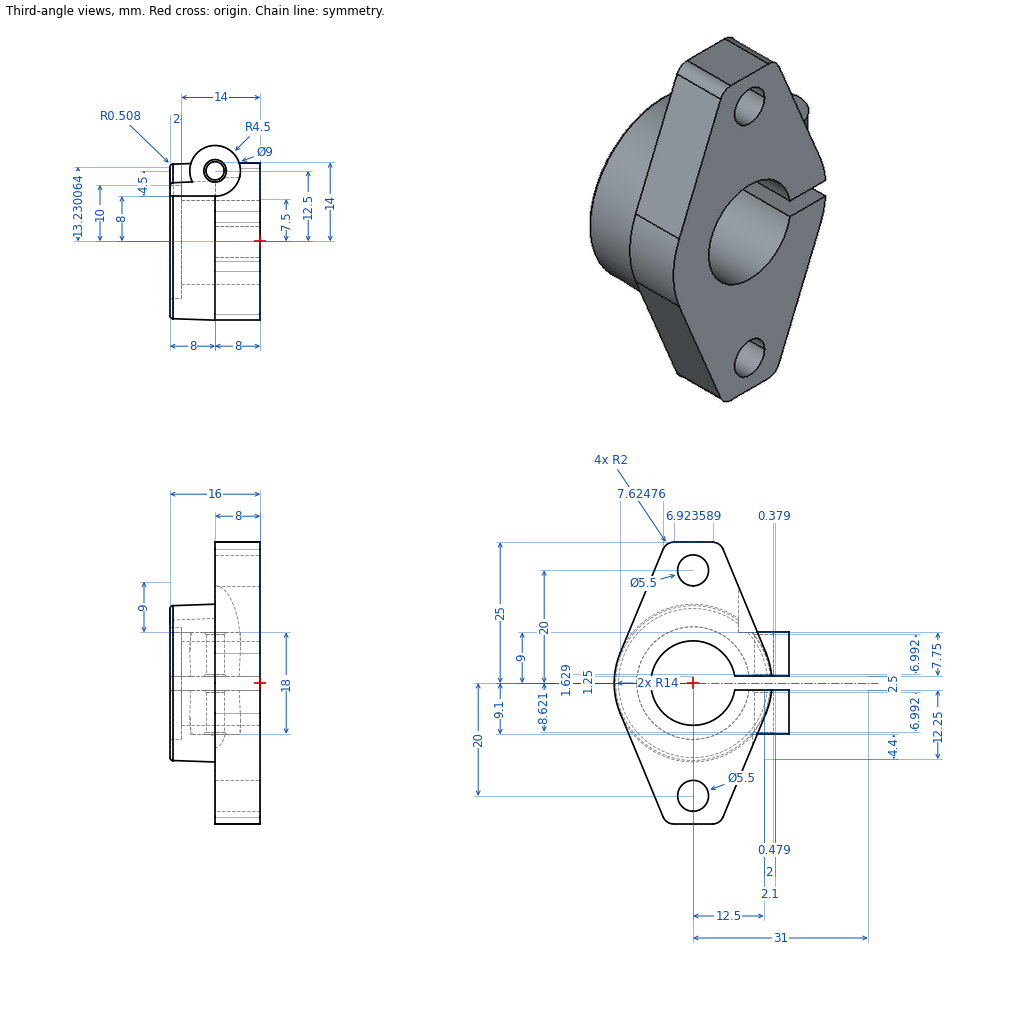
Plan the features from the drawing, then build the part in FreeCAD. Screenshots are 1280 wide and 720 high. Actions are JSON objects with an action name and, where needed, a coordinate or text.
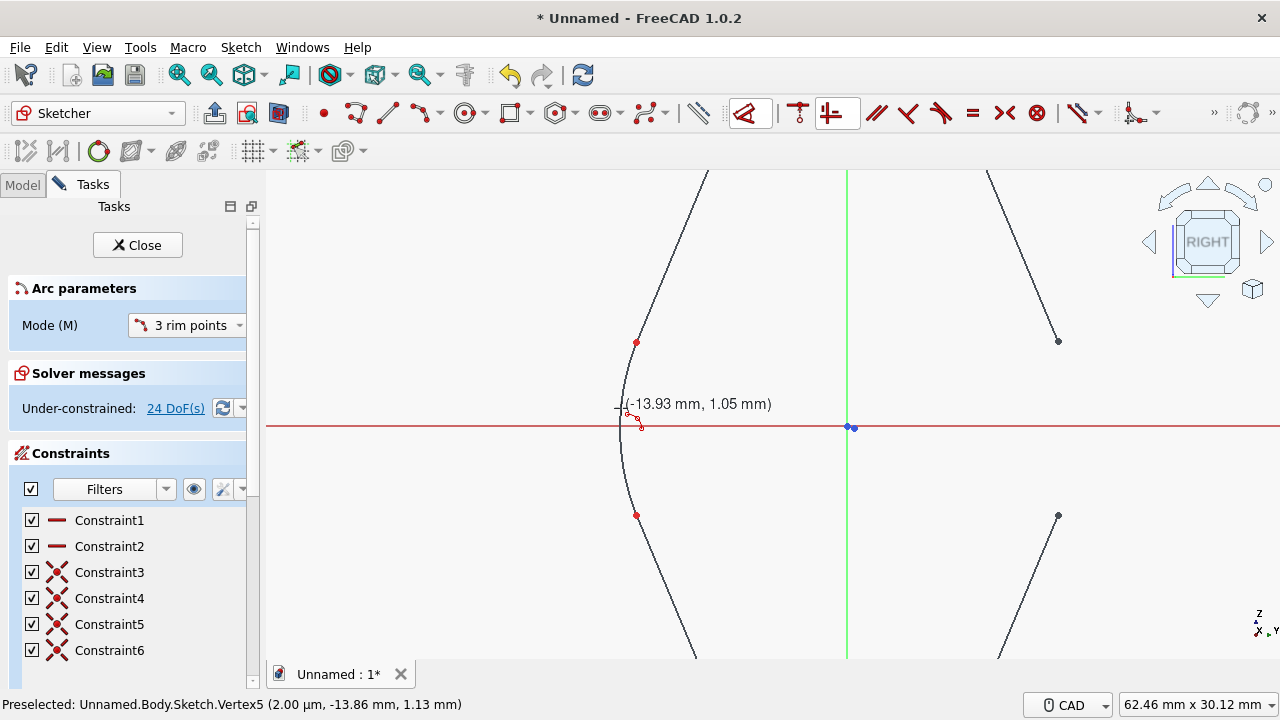
{"action": "scroll", "coordinate": [621, 408], "scroll_direction": "down", "scroll_amount": 5}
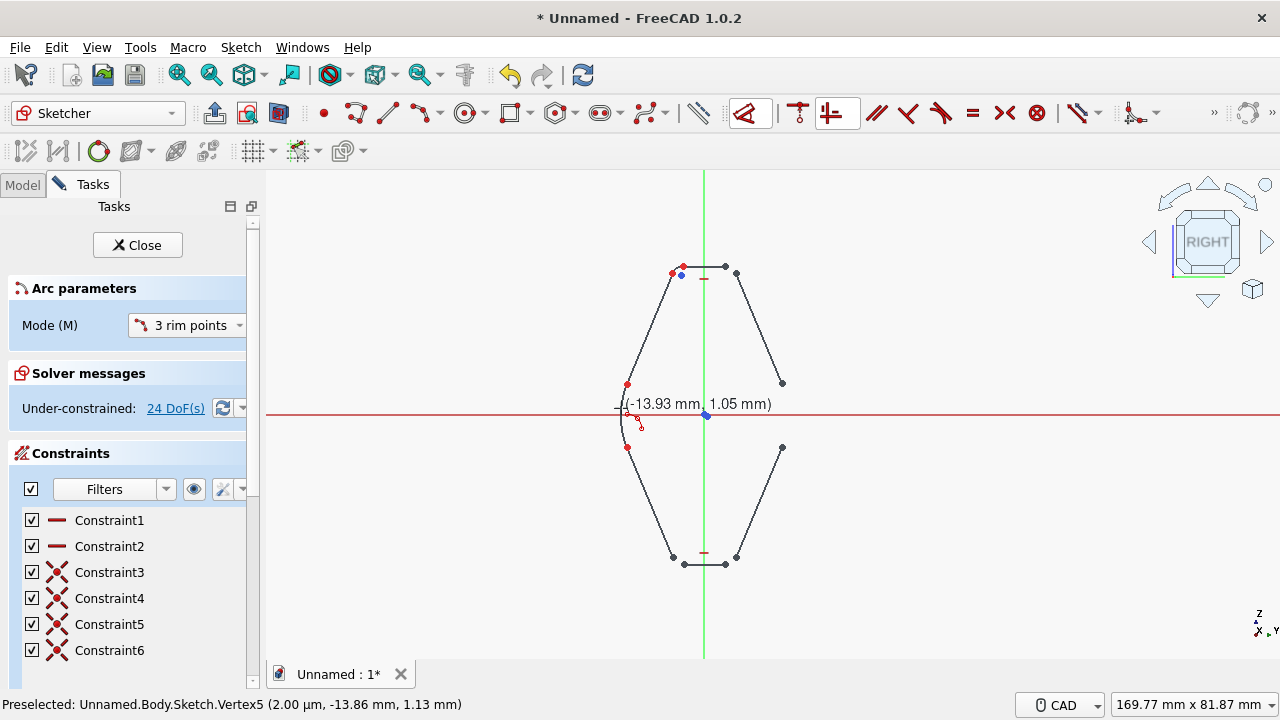
{"action": "left_click", "coordinate": [673, 558]}
{"action": "left_click", "coordinate": [684, 565]}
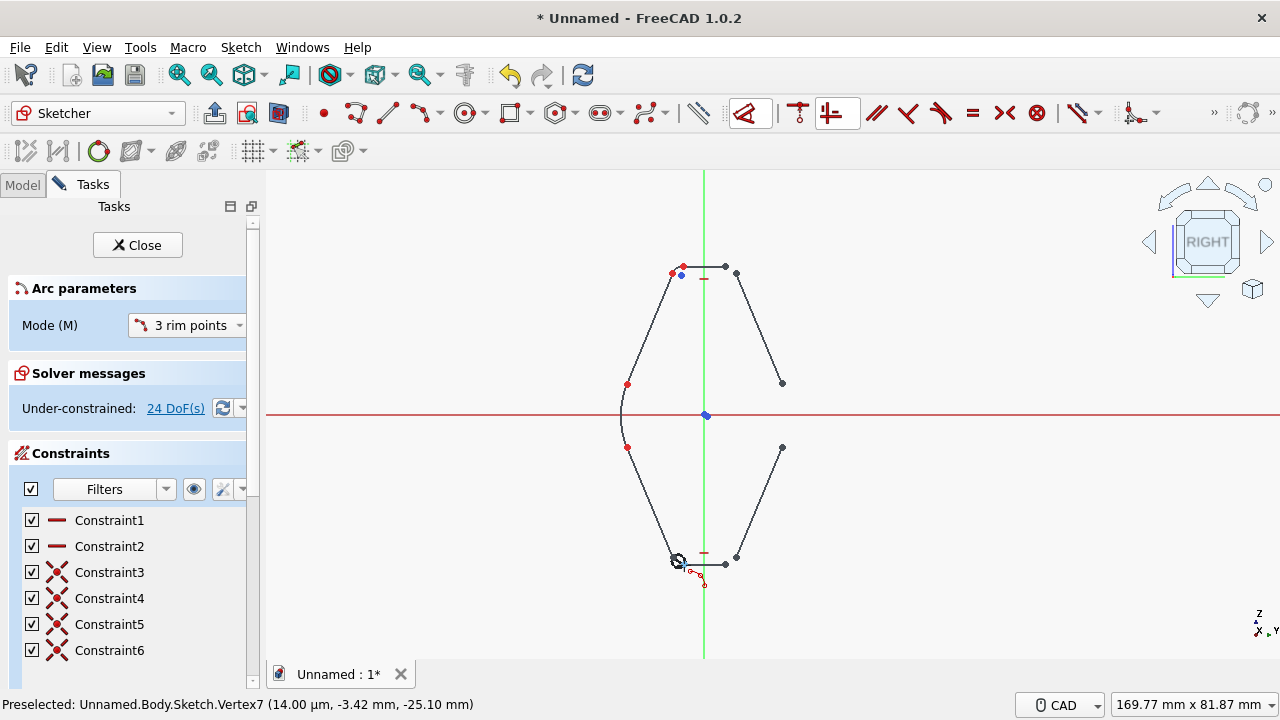
{"action": "scroll", "coordinate": [677, 562], "scroll_direction": "up", "scroll_amount": 11}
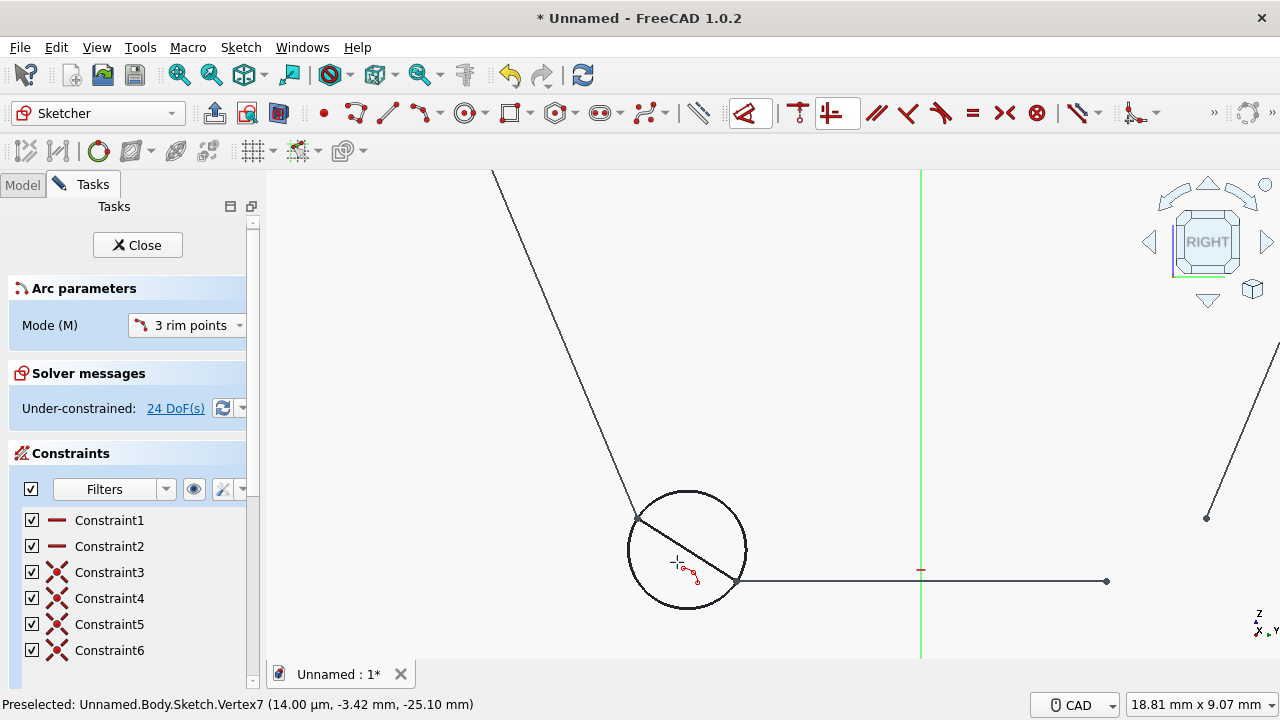
{"action": "left_click", "coordinate": [675, 558]}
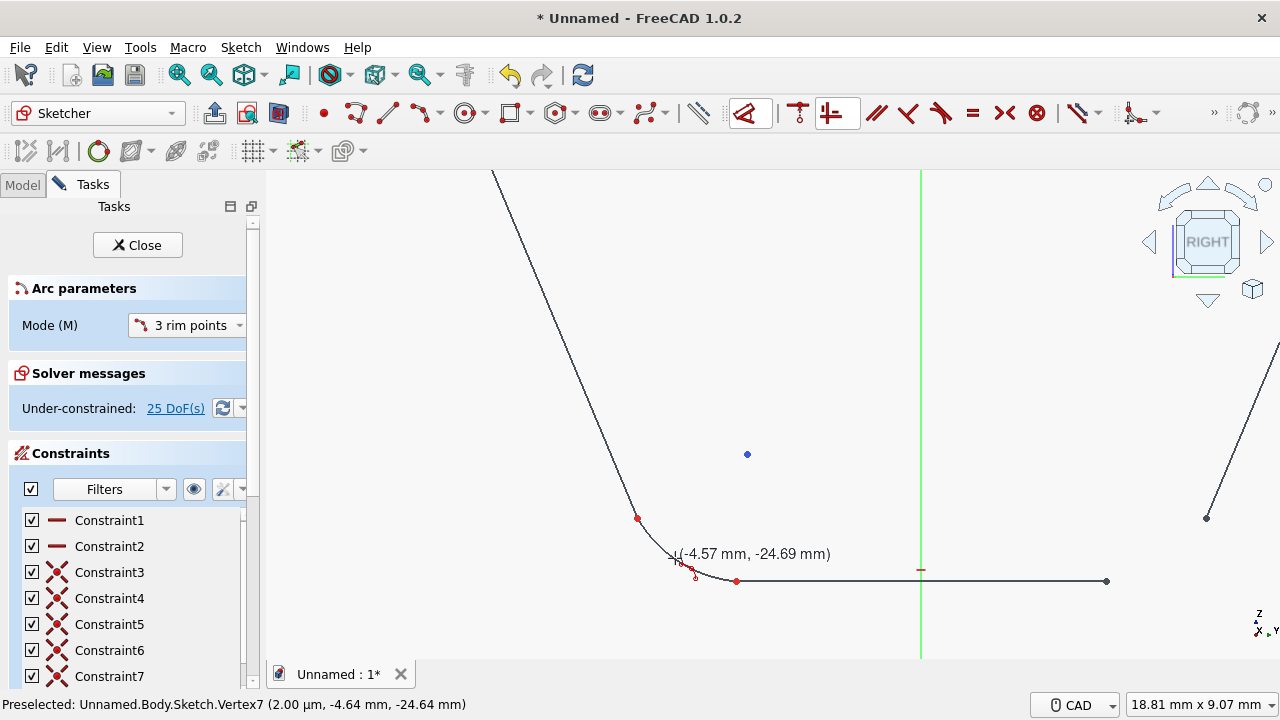
{"action": "scroll", "coordinate": [677, 562], "scroll_direction": "down", "scroll_amount": 11}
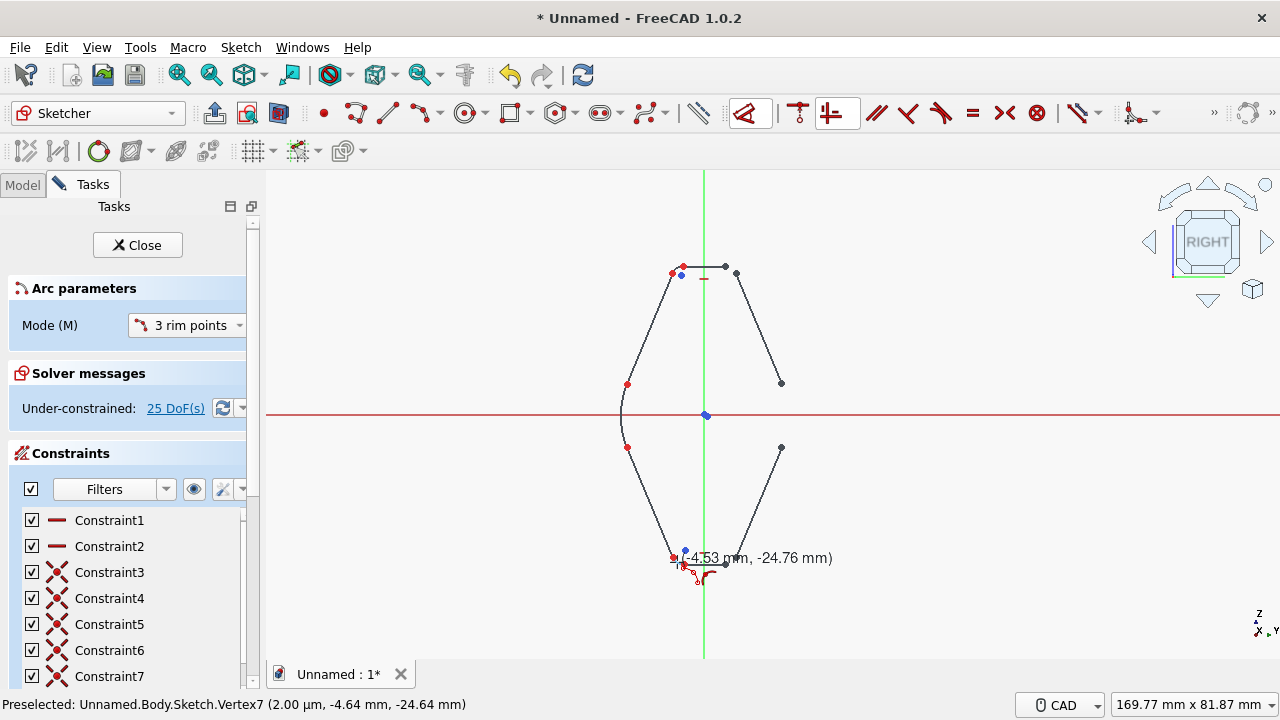
{"action": "left_click", "coordinate": [725, 565]}
{"action": "left_click", "coordinate": [736, 558]}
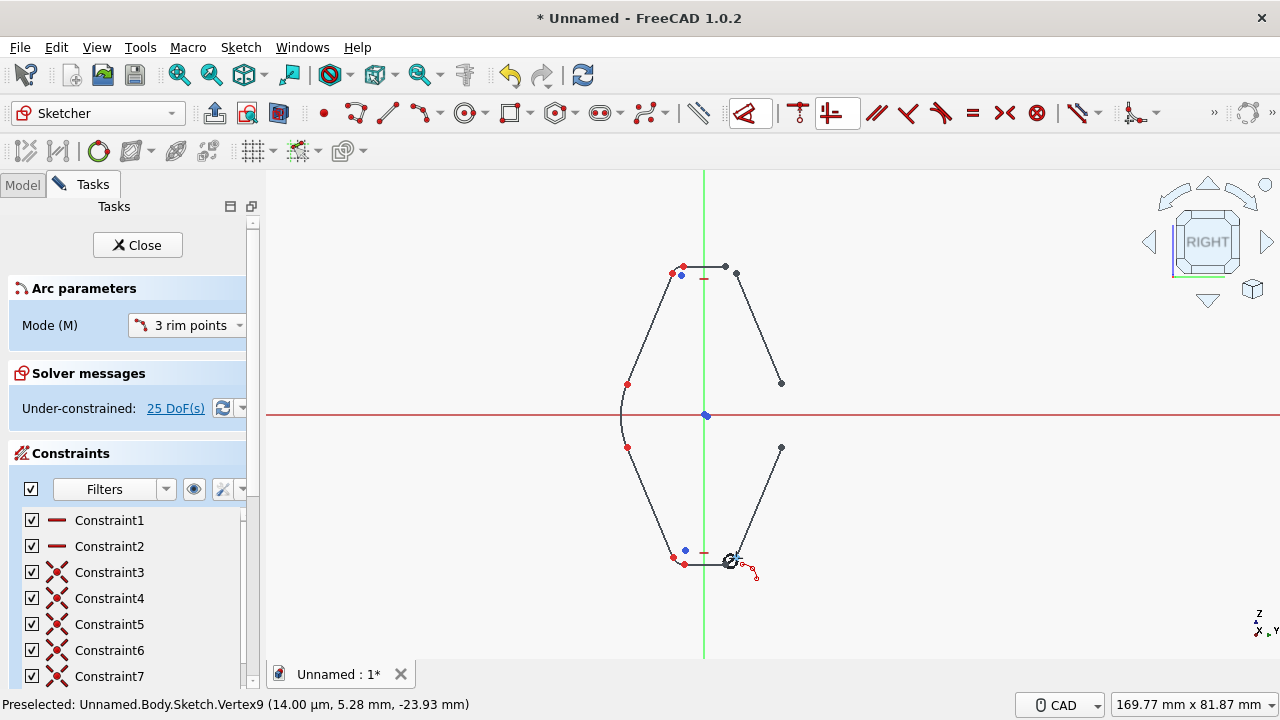
{"action": "scroll", "coordinate": [732, 562], "scroll_direction": "up", "scroll_amount": 11}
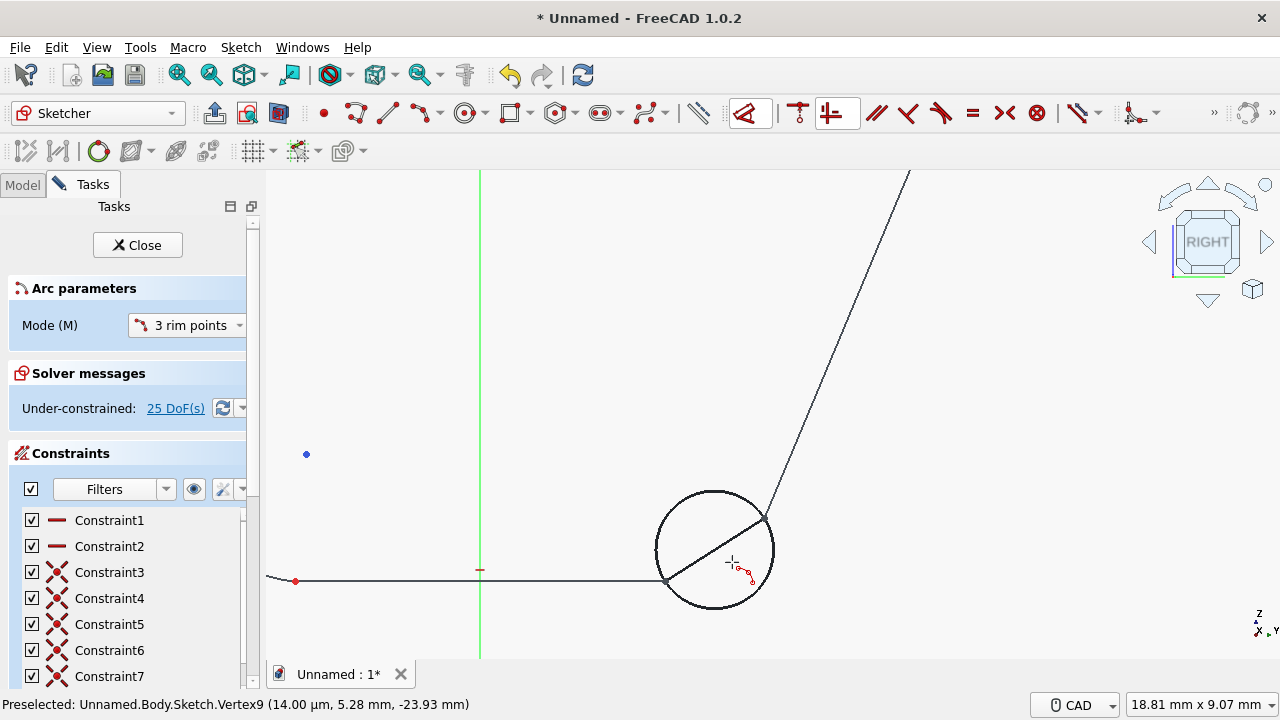
{"action": "left_click", "coordinate": [726, 558]}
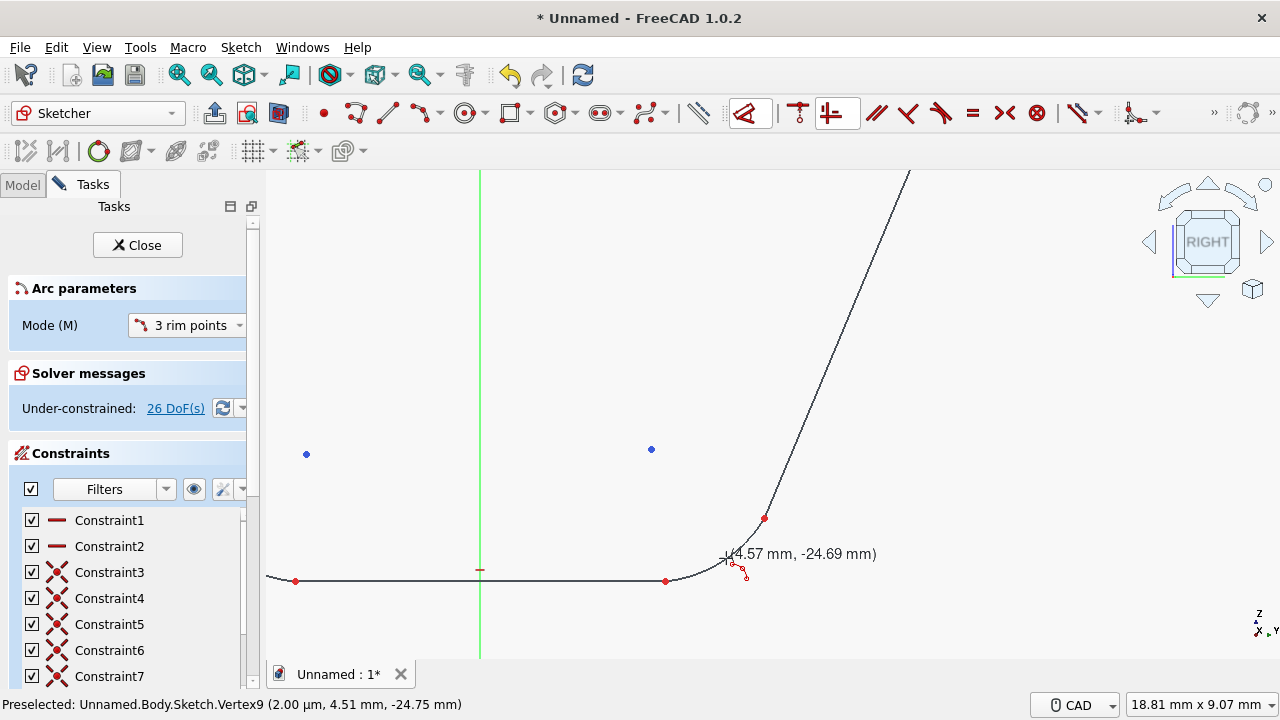
{"action": "scroll", "coordinate": [733, 562], "scroll_direction": "down", "scroll_amount": 11}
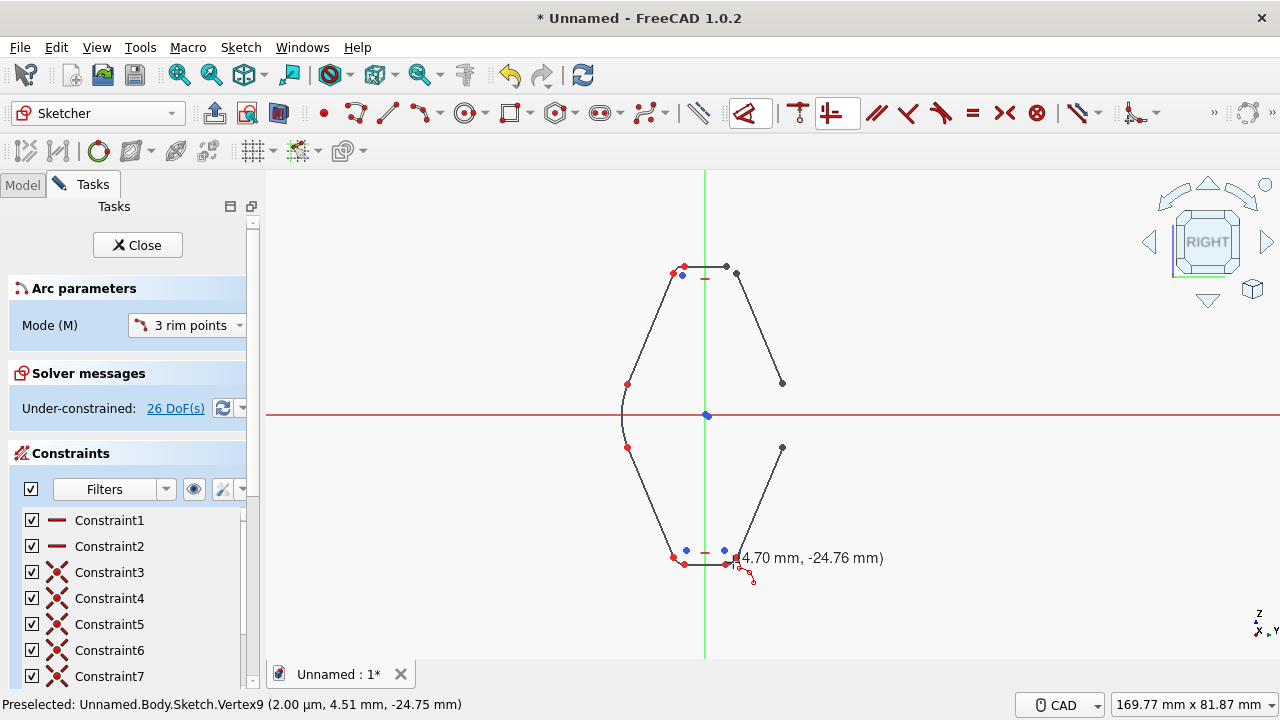
{"action": "left_click", "coordinate": [783, 448]}
{"action": "left_click", "coordinate": [783, 384]}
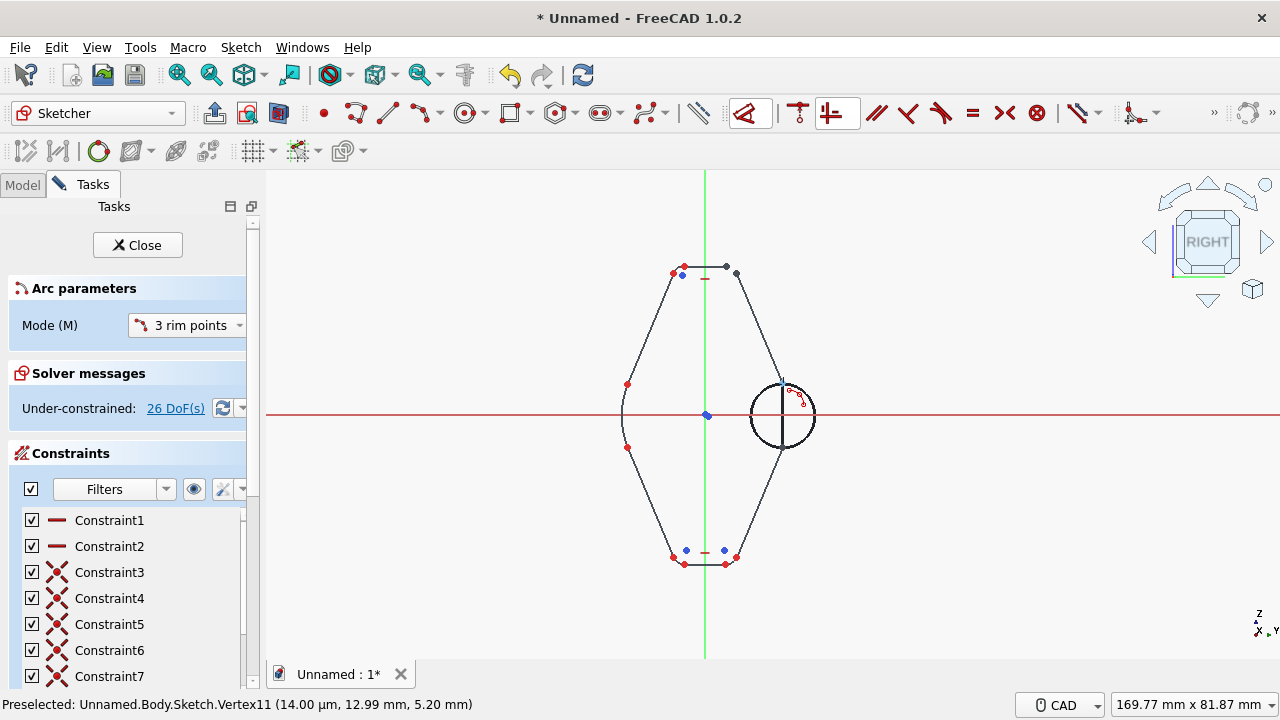
{"action": "scroll", "coordinate": [789, 422], "scroll_direction": "up", "scroll_amount": 5}